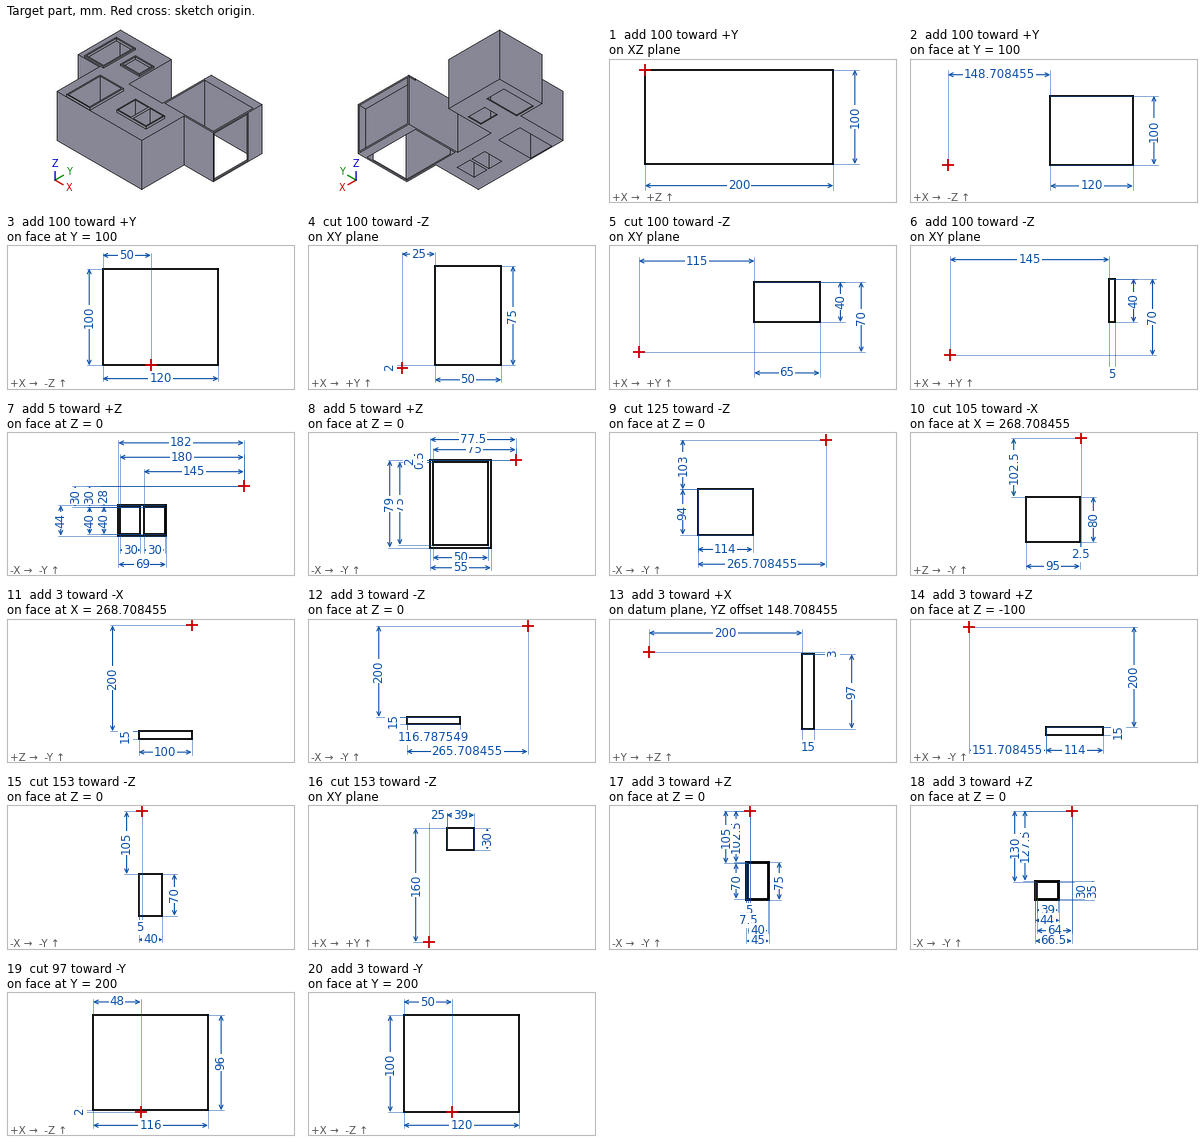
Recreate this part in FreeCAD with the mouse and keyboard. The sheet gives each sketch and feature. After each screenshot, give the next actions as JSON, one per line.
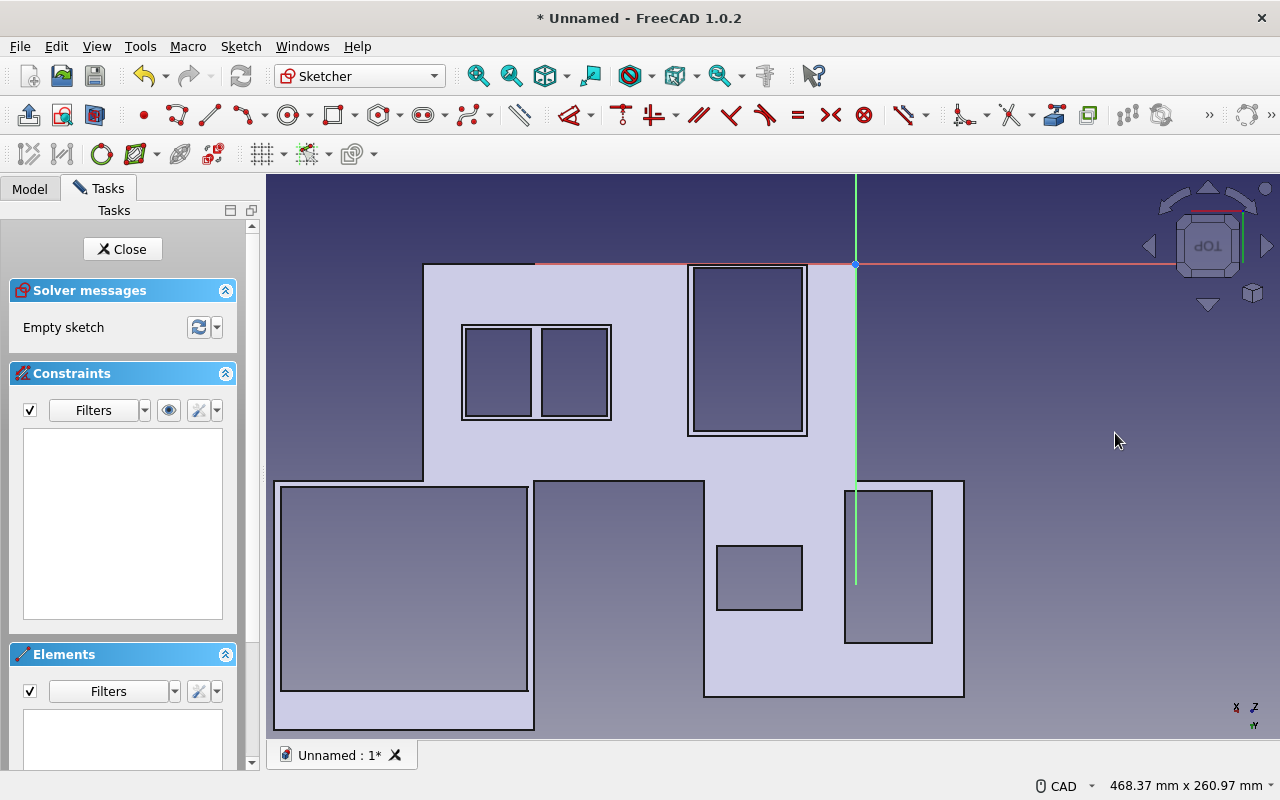
{"action": "left_click", "coordinate": [332, 116]}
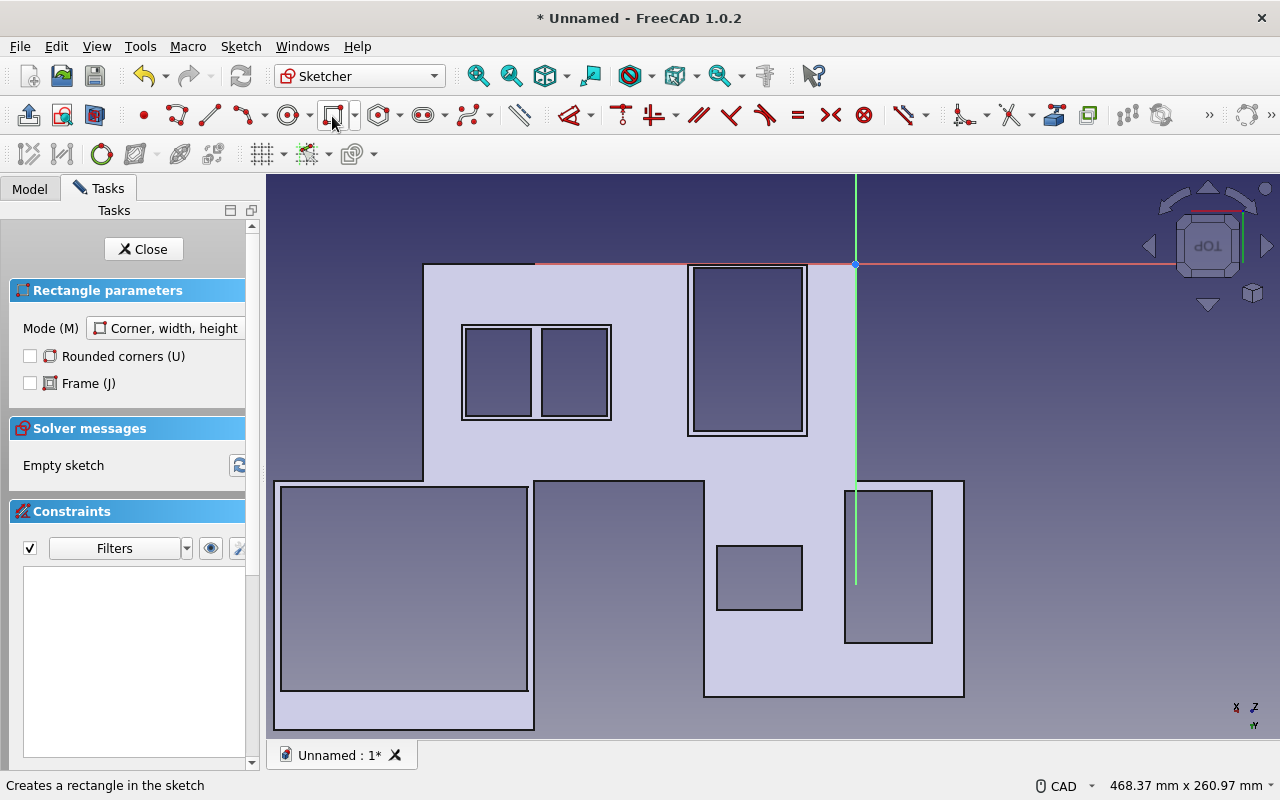
{"action": "left_click", "coordinate": [840, 486]}
{"action": "mouse_move", "coordinate": [937, 648]}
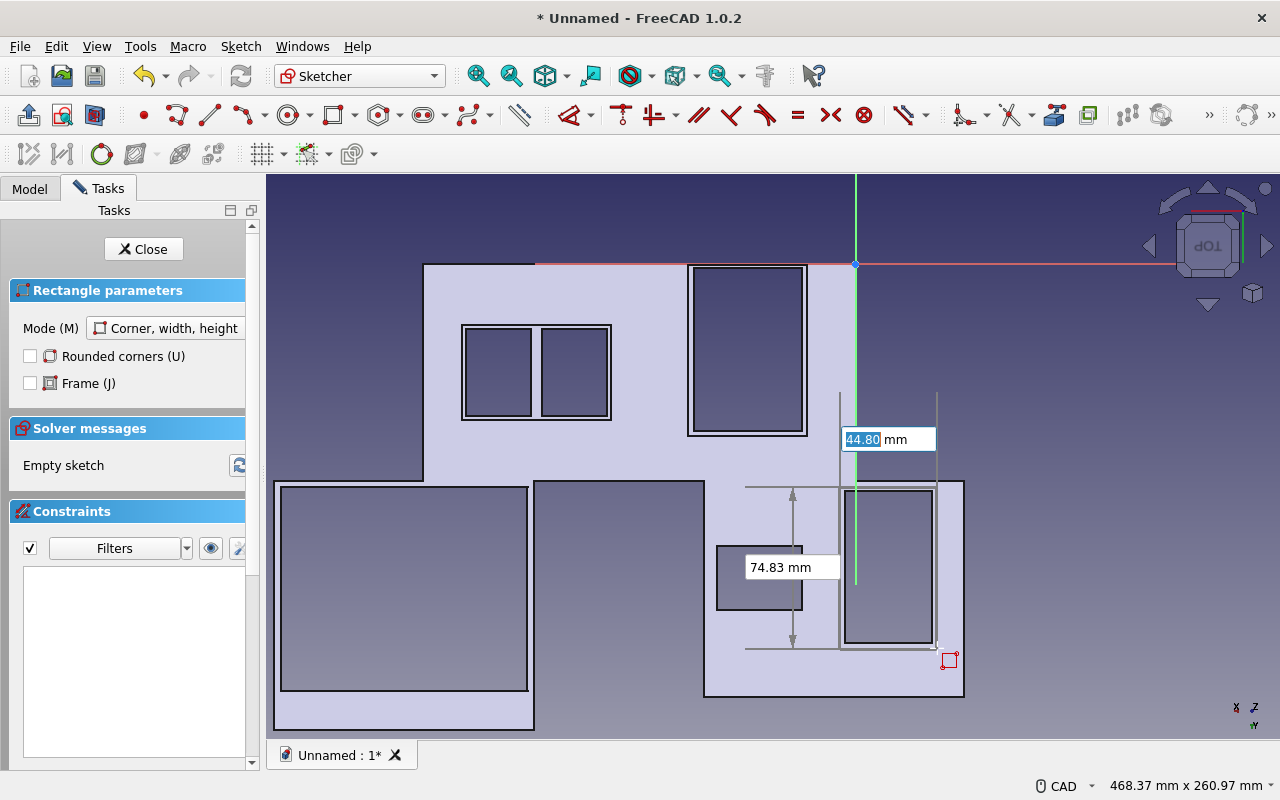
{"action": "type", "text": "45"}
{"action": "key", "text": "Tab"}
{"action": "type", "text": "75"}
{"action": "key", "text": "Return"}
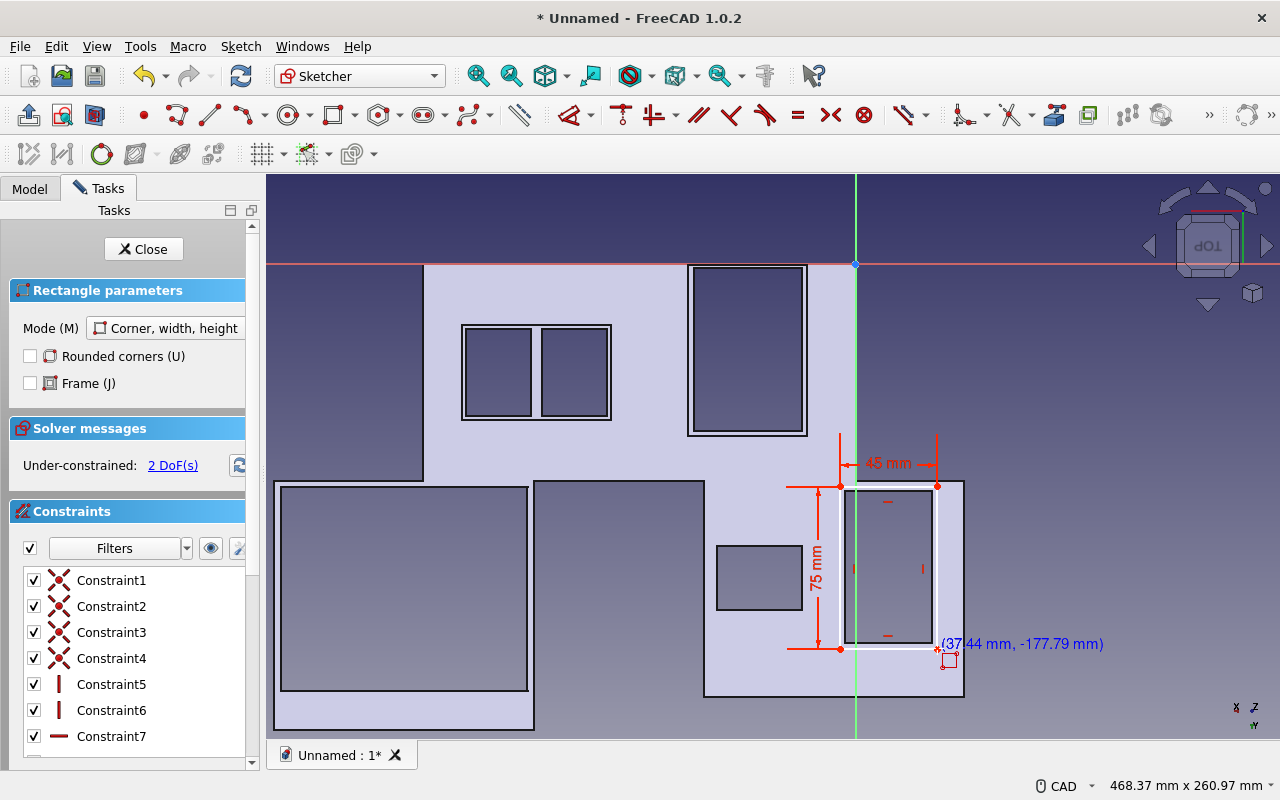
{"action": "scroll", "coordinate": [845, 491], "scroll_direction": "up", "scroll_amount": 6}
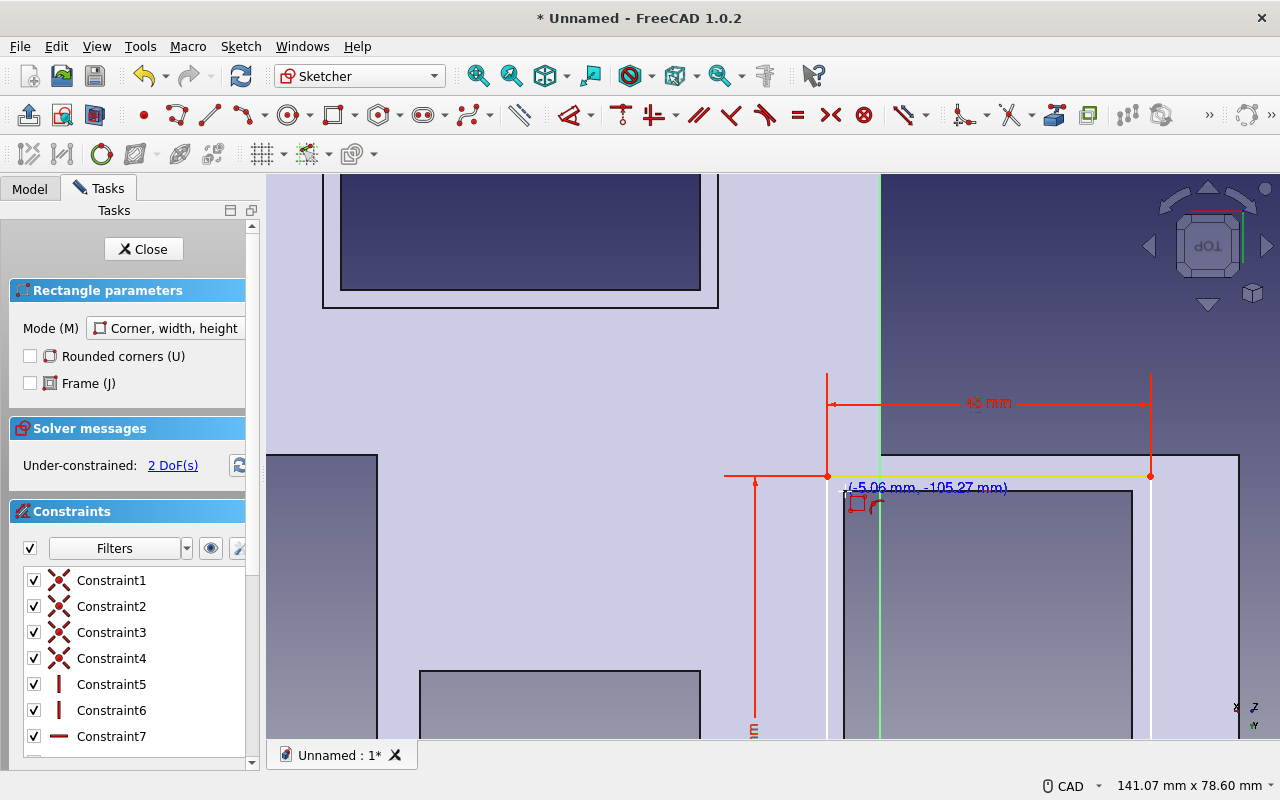
{"action": "left_click", "coordinate": [844, 491]}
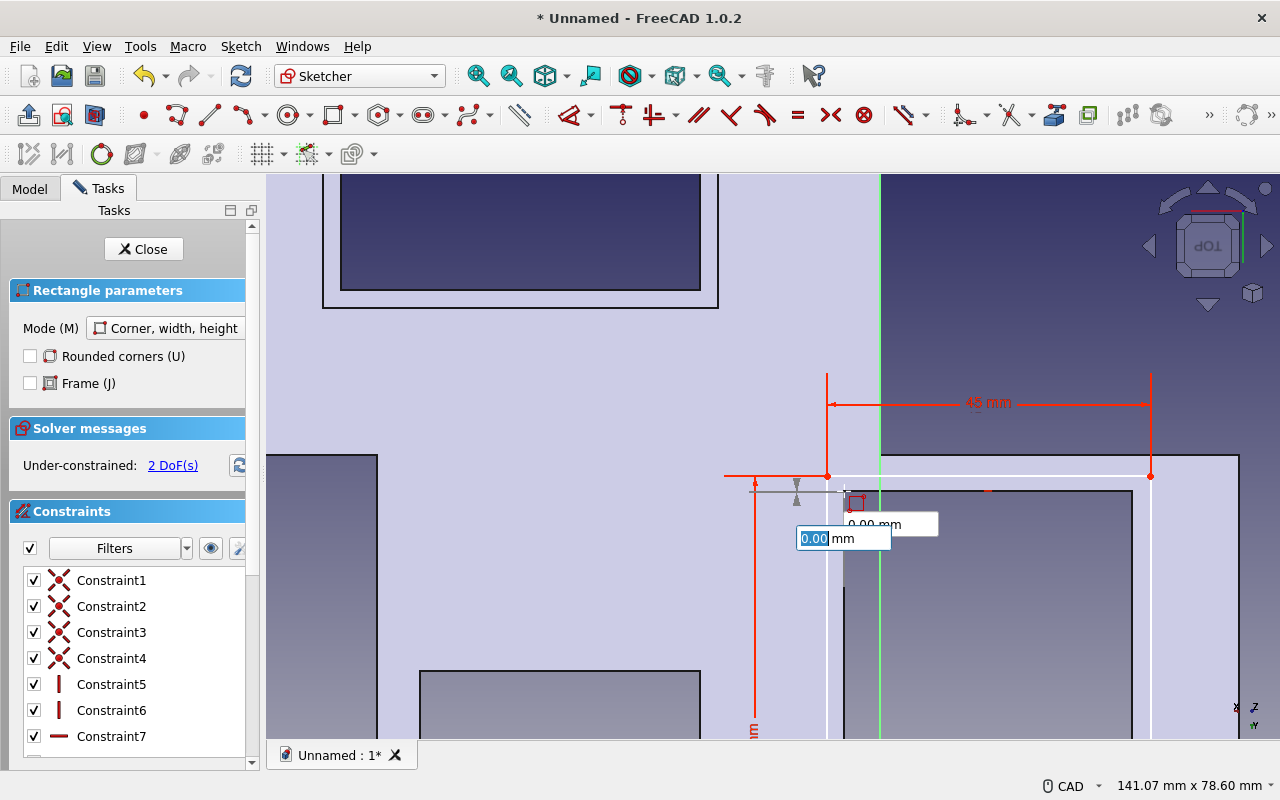
{"action": "scroll", "coordinate": [582, 492], "scroll_direction": "down", "scroll_amount": 6}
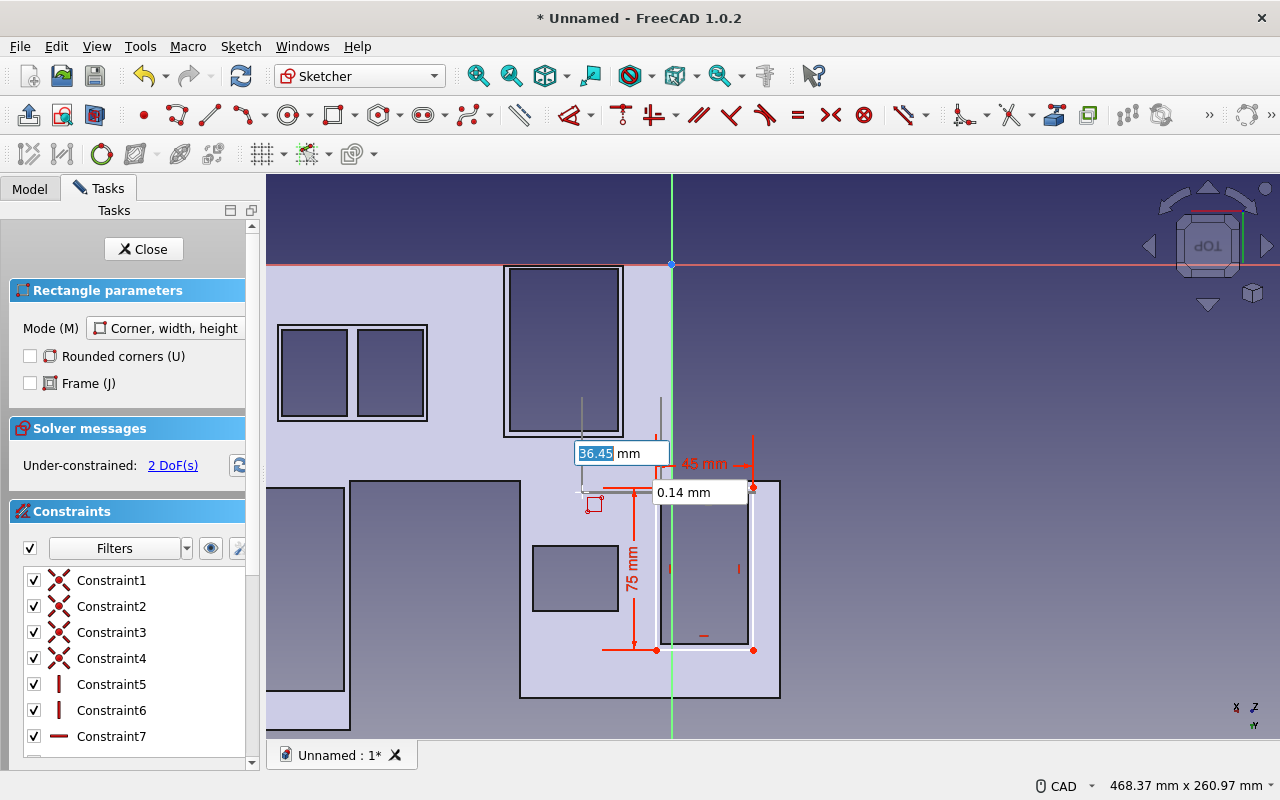
{"action": "scroll", "coordinate": [748, 644], "scroll_direction": "up", "scroll_amount": 6}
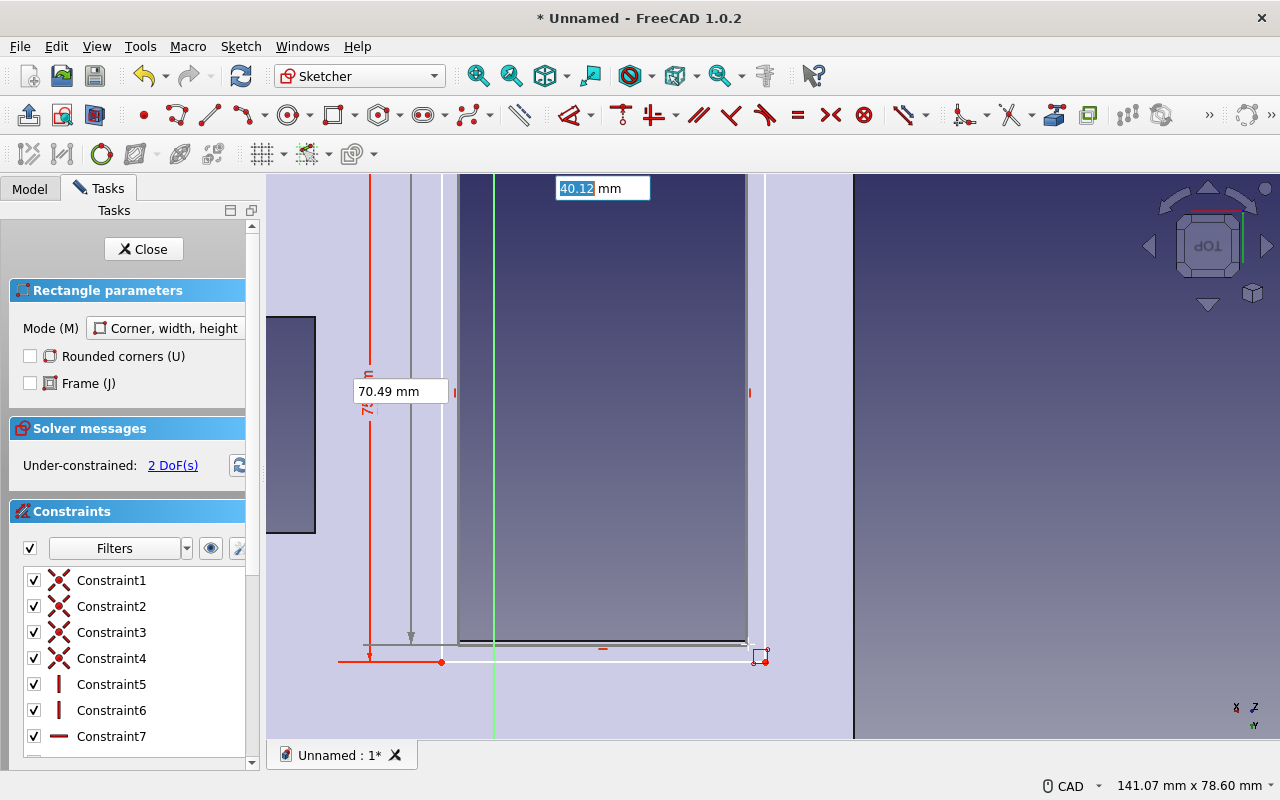
{"action": "left_click", "coordinate": [746, 641]}
{"action": "key", "text": "Escape"}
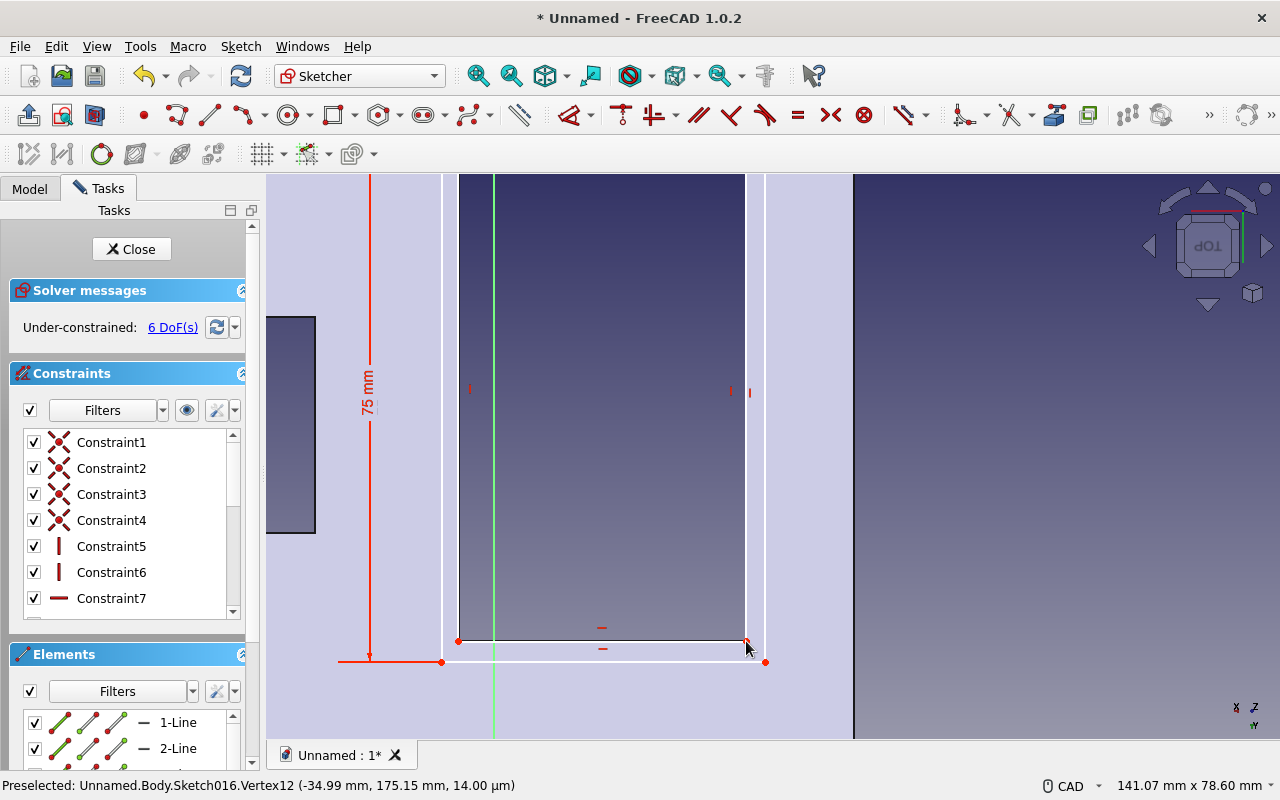
{"action": "left_click", "coordinate": [568, 116]}